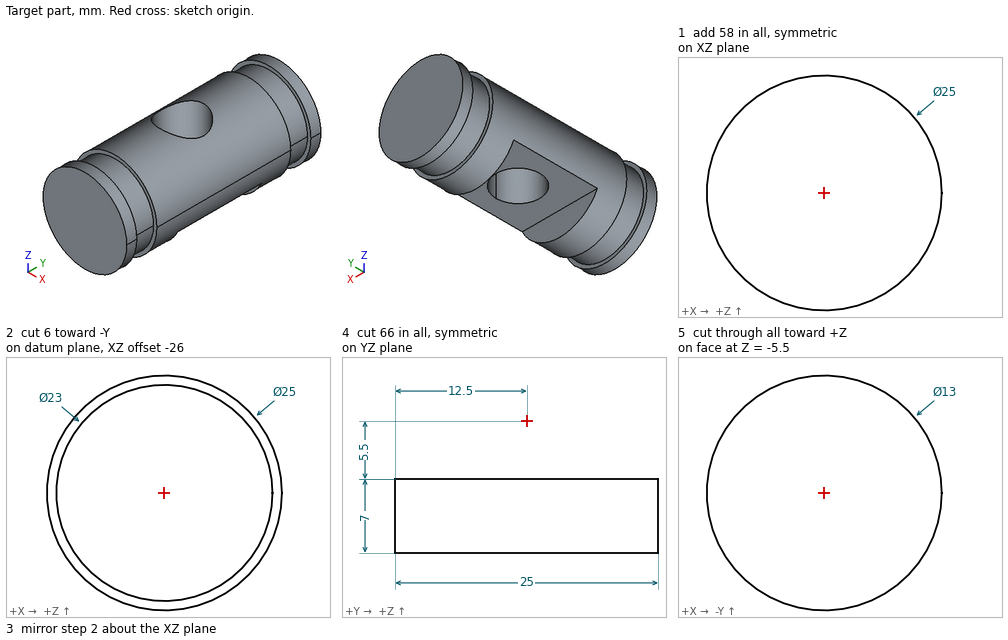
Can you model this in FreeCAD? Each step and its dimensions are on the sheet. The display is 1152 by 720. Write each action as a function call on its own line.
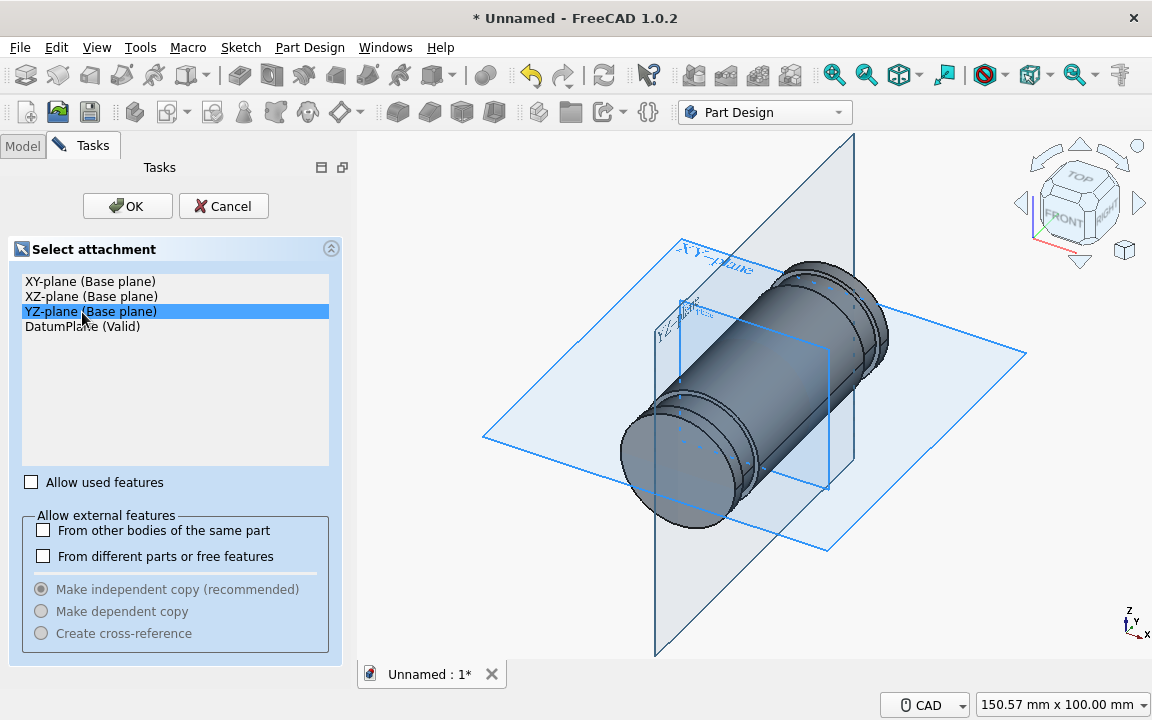
click(128, 206)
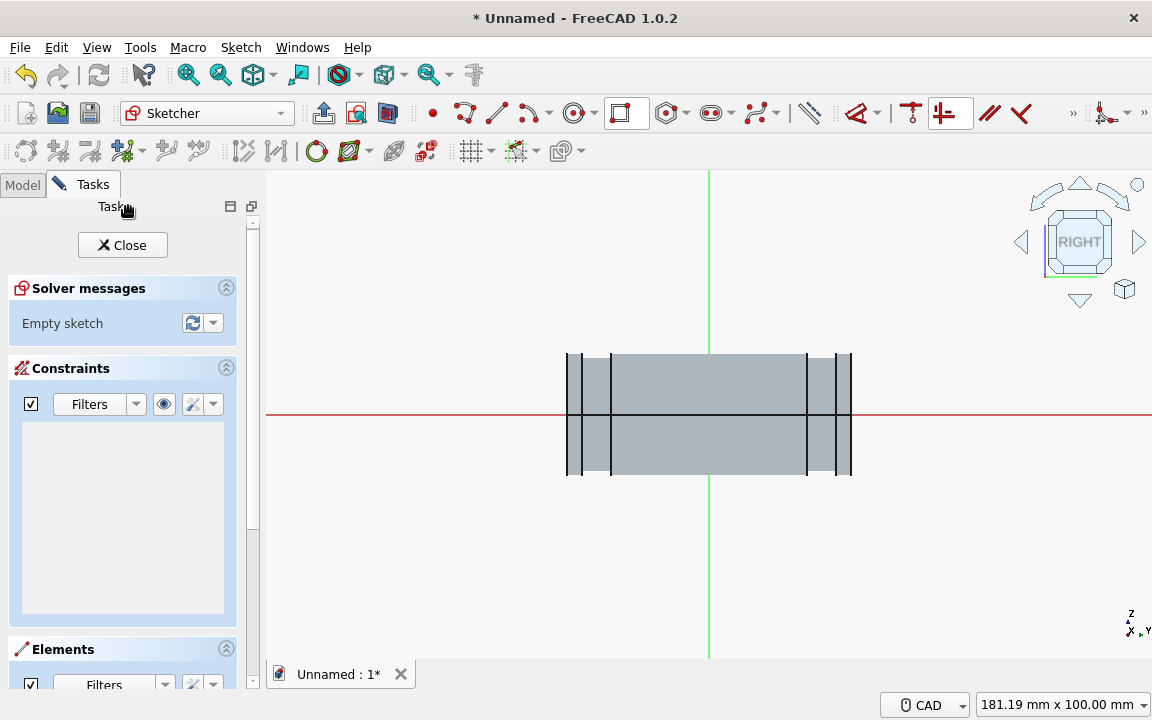
click(388, 114)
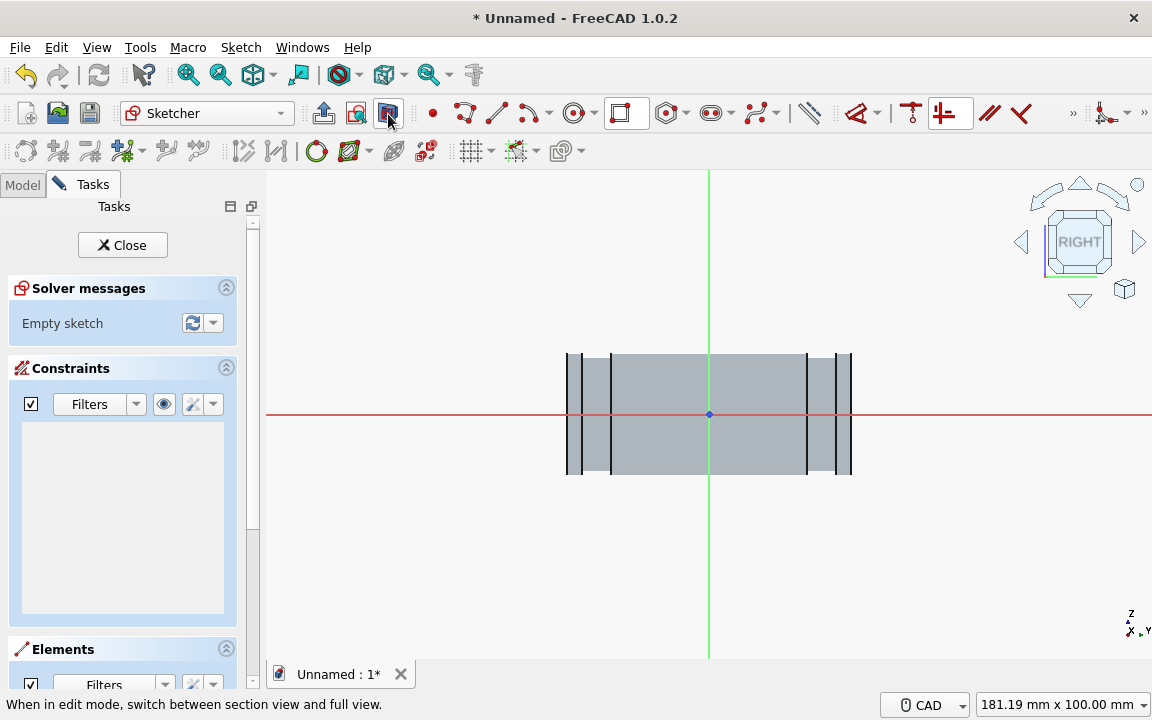
scroll(731, 455, up, 7)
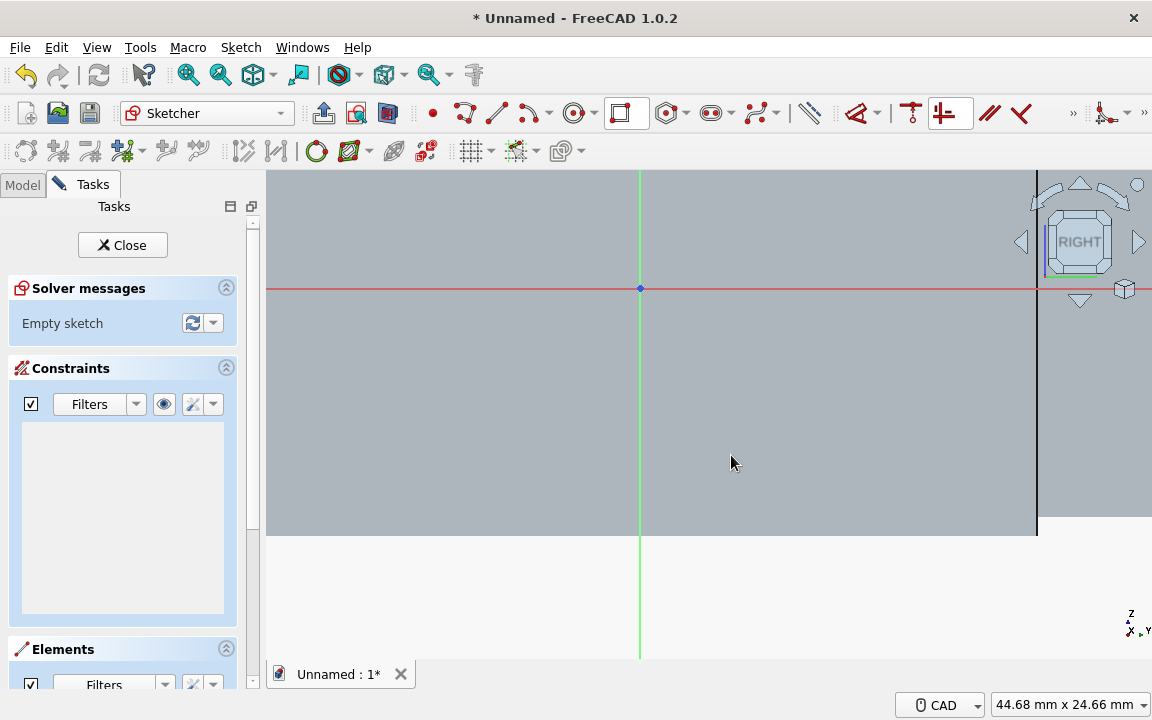
click(620, 114)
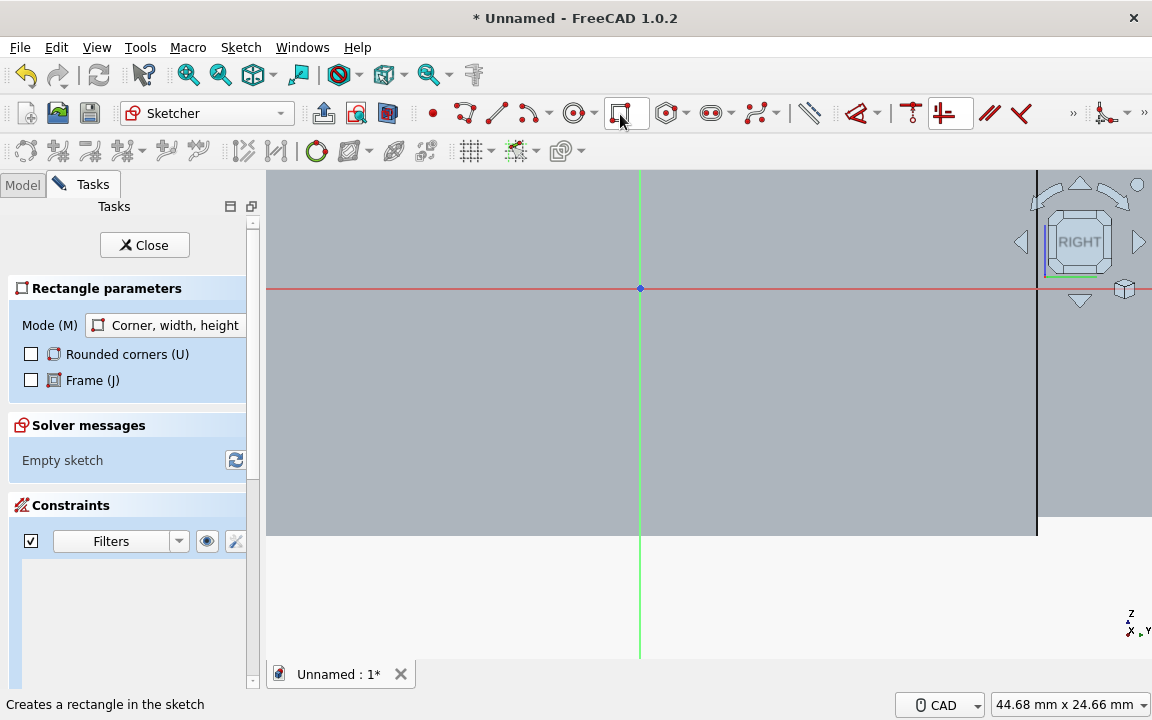
click(392, 398)
click(888, 537)
key(Escape)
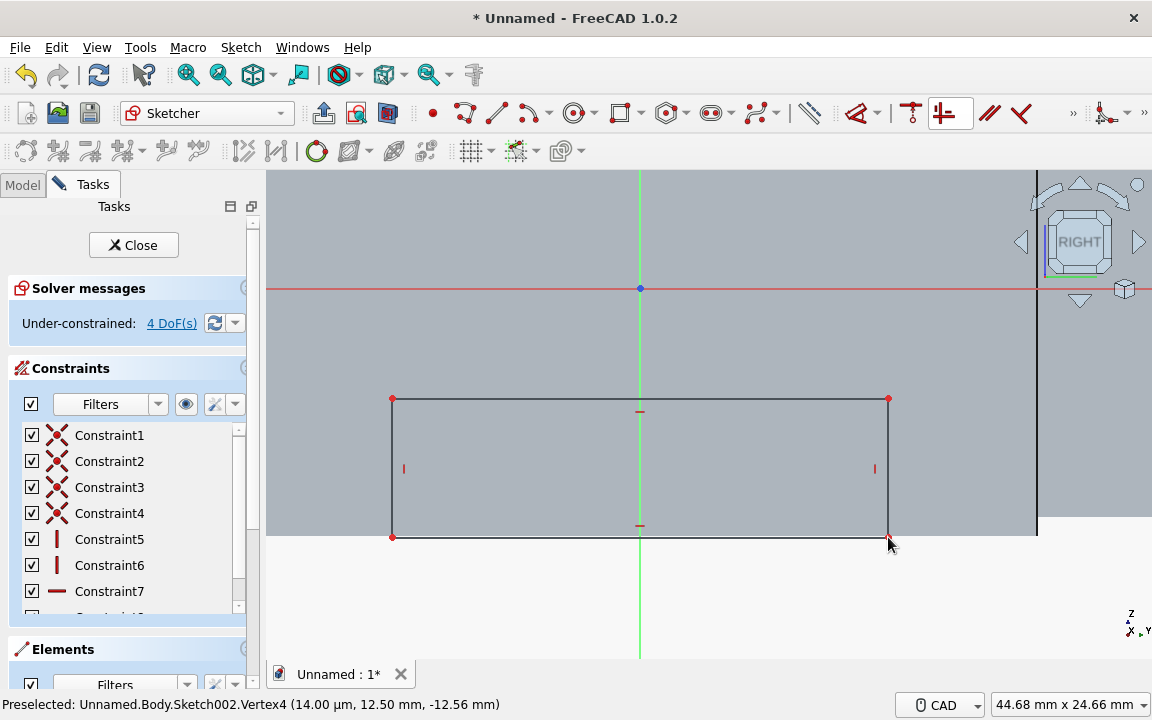
click(856, 114)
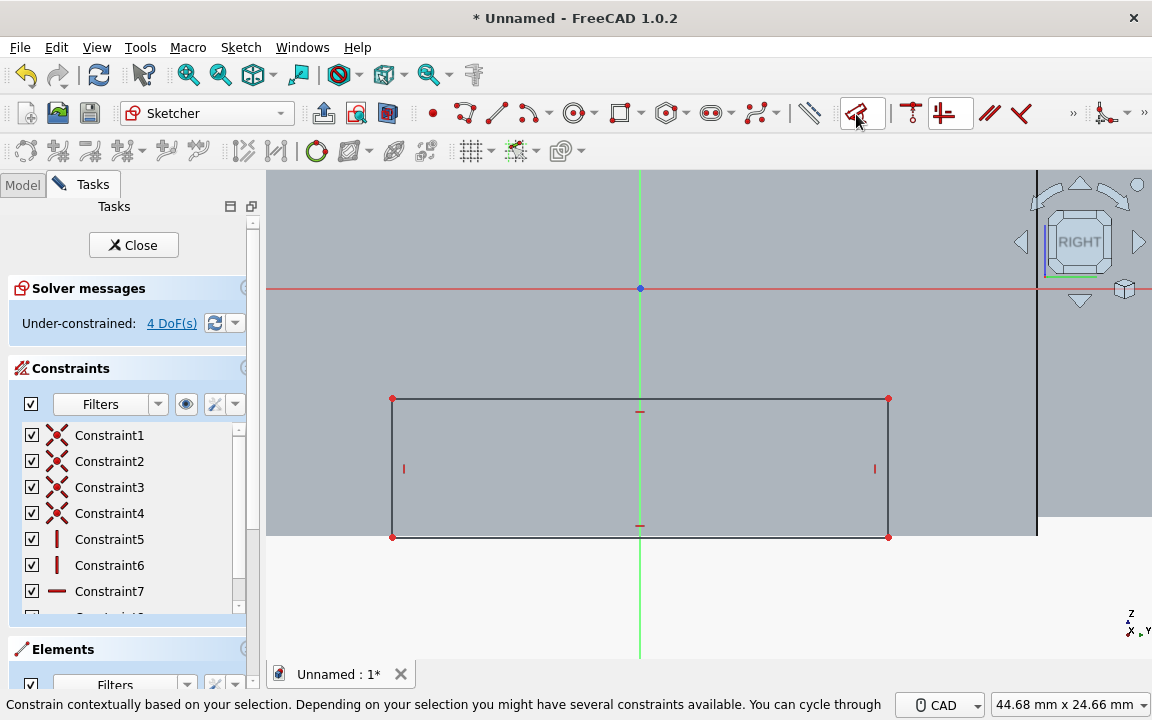
click(392, 441)
click(358, 469)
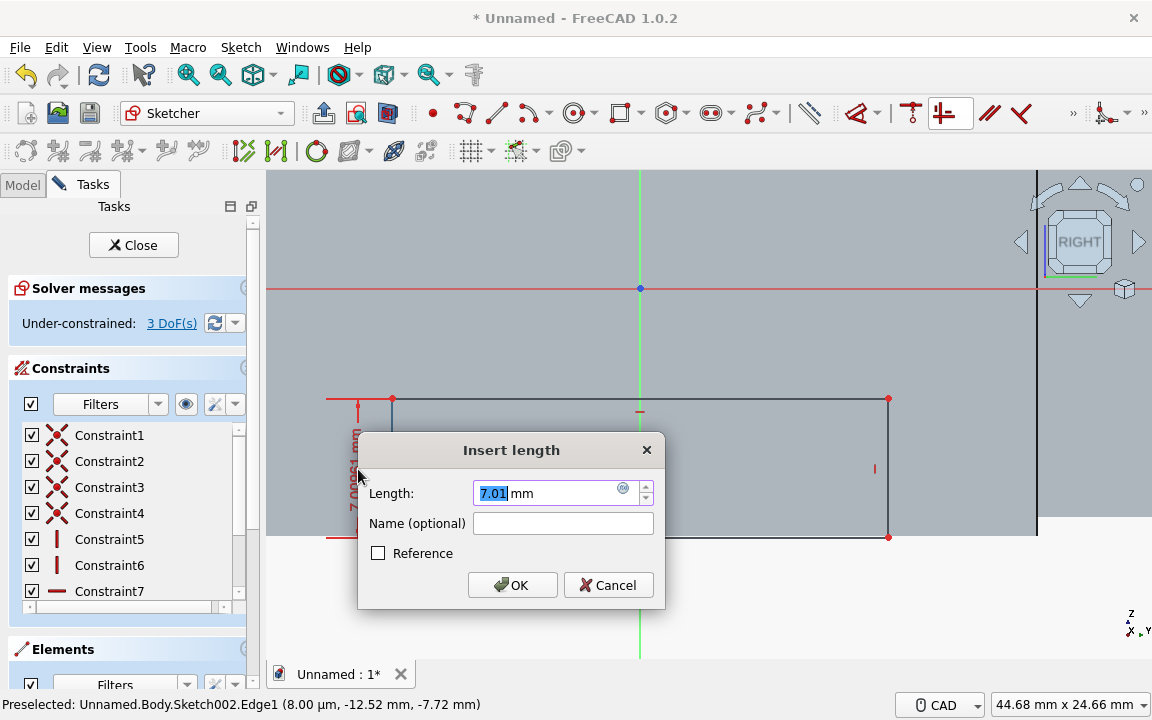
text(7)
key(Return)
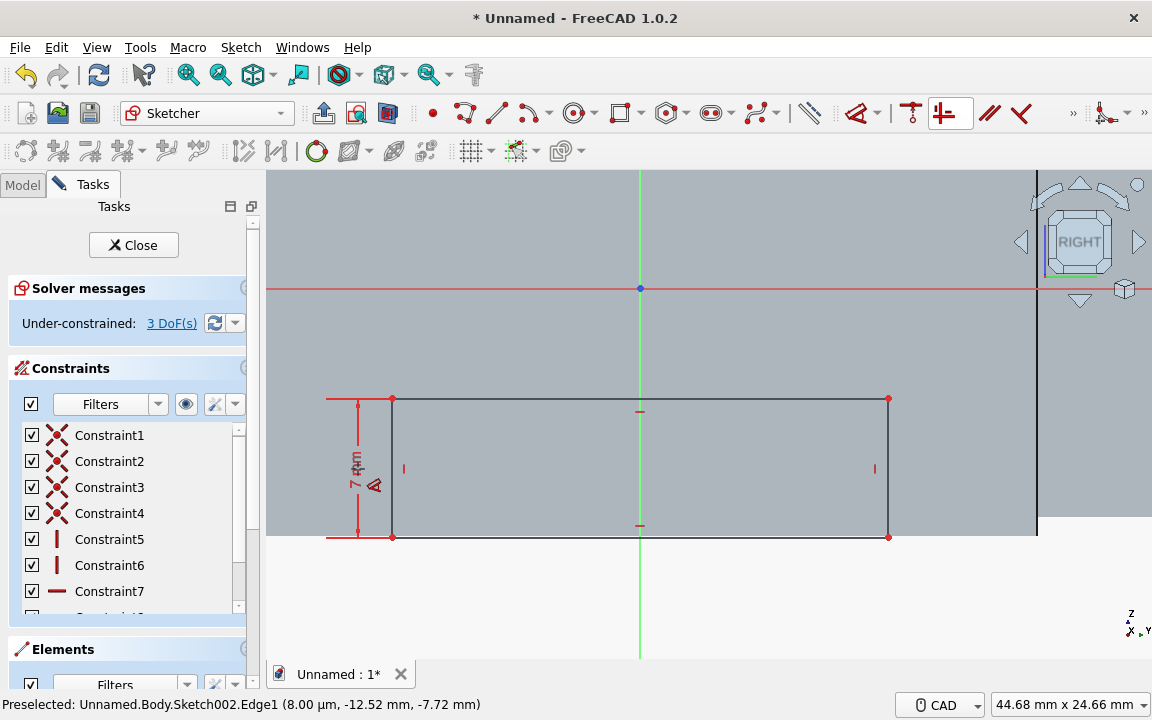
click(541, 538)
click(526, 572)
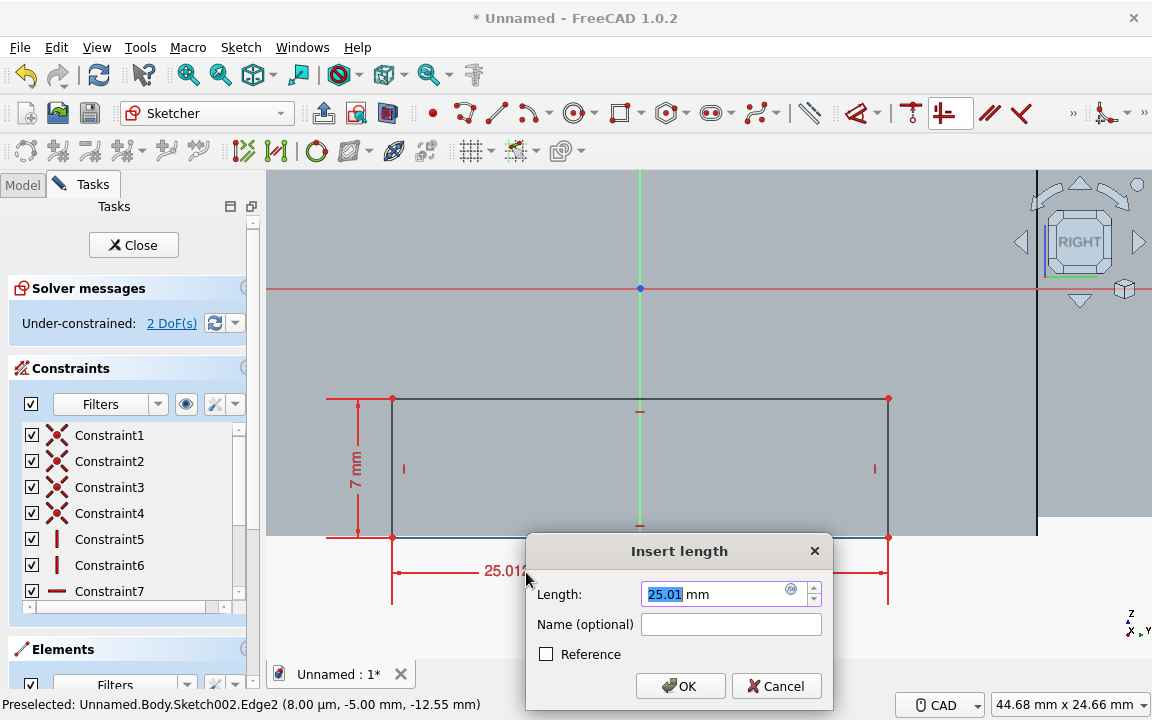
text(25)
key(Return)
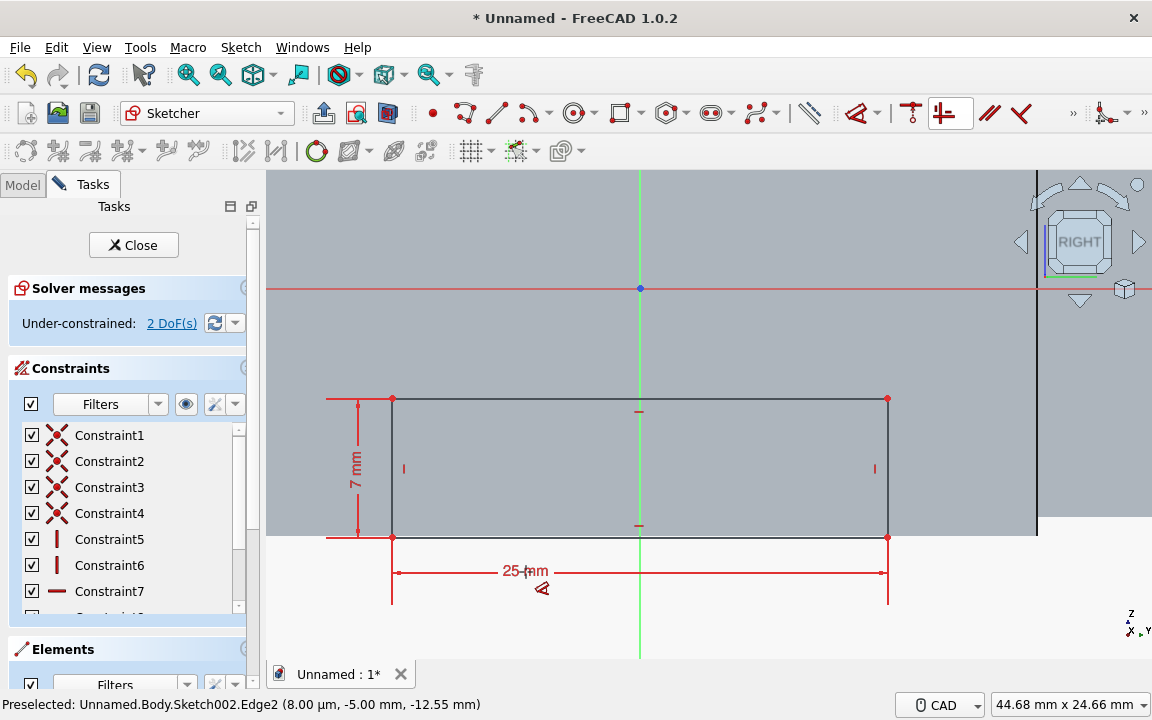
click(392, 399)
click(358, 344)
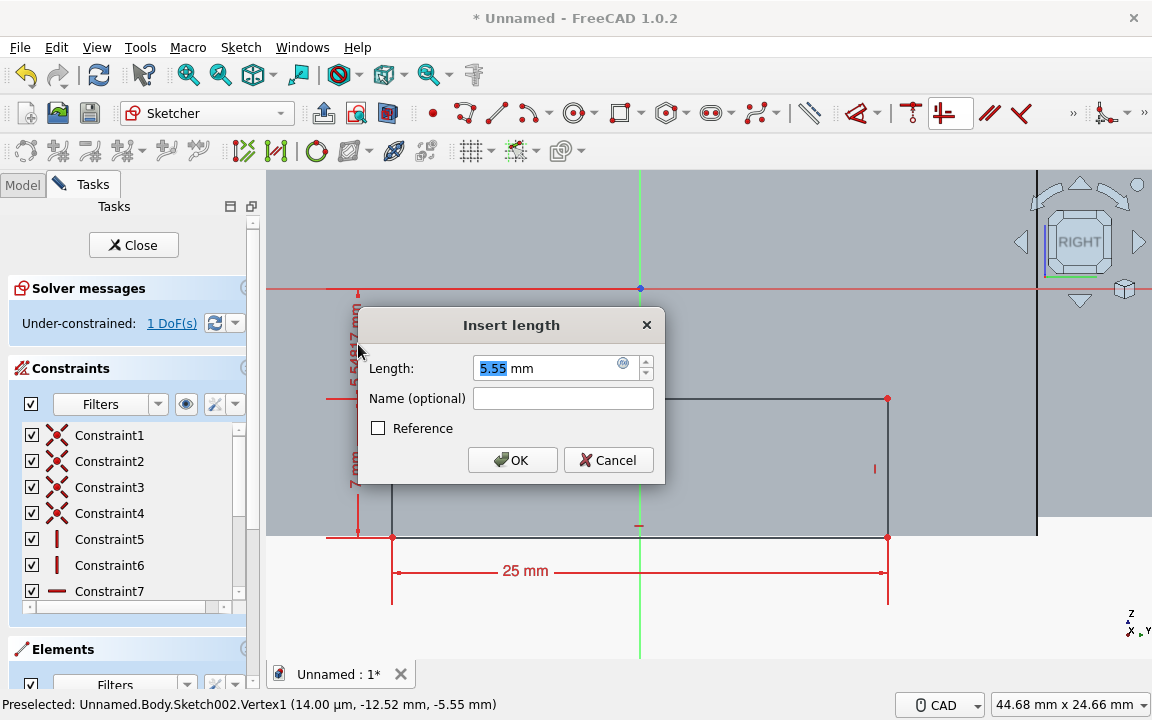
text(5.5)
key(Return)